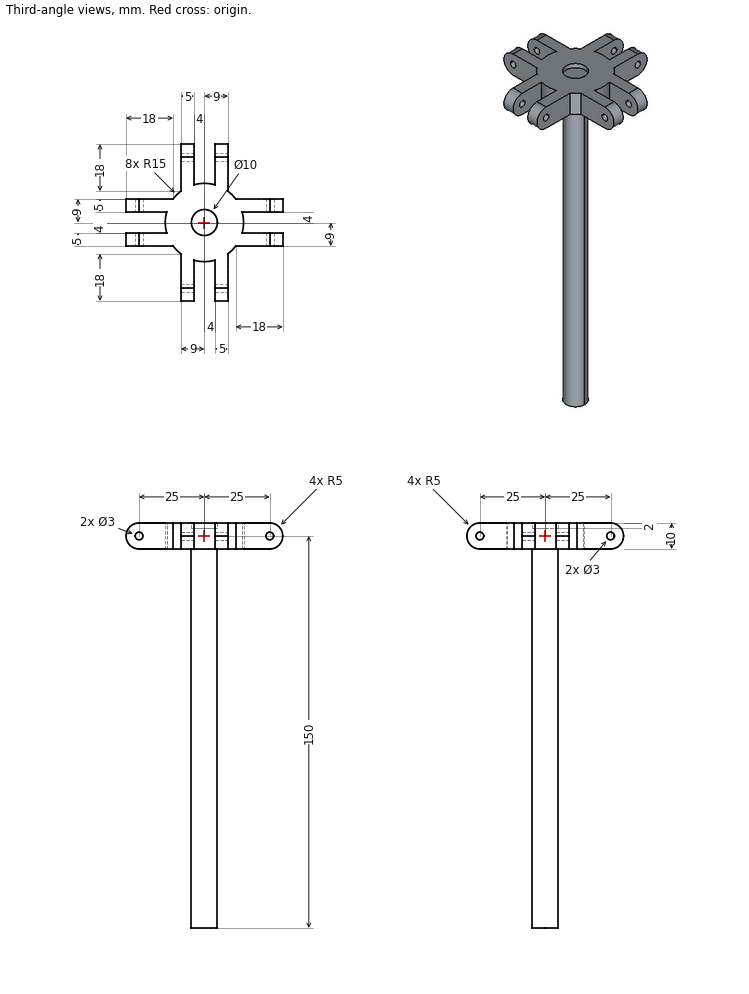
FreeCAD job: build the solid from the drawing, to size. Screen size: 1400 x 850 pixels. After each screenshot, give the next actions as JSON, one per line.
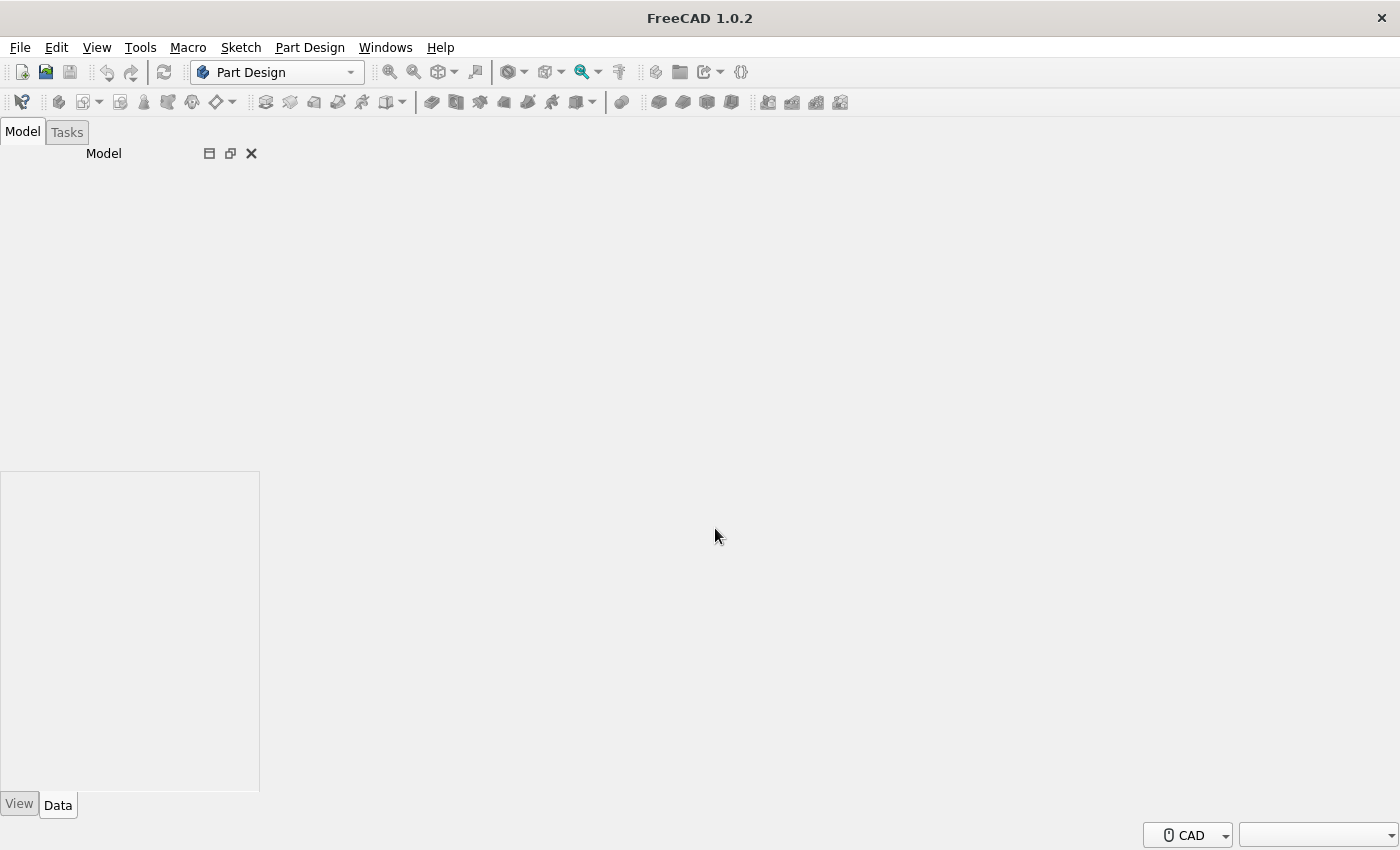
{"action": "left_click", "coordinate": [22, 72]}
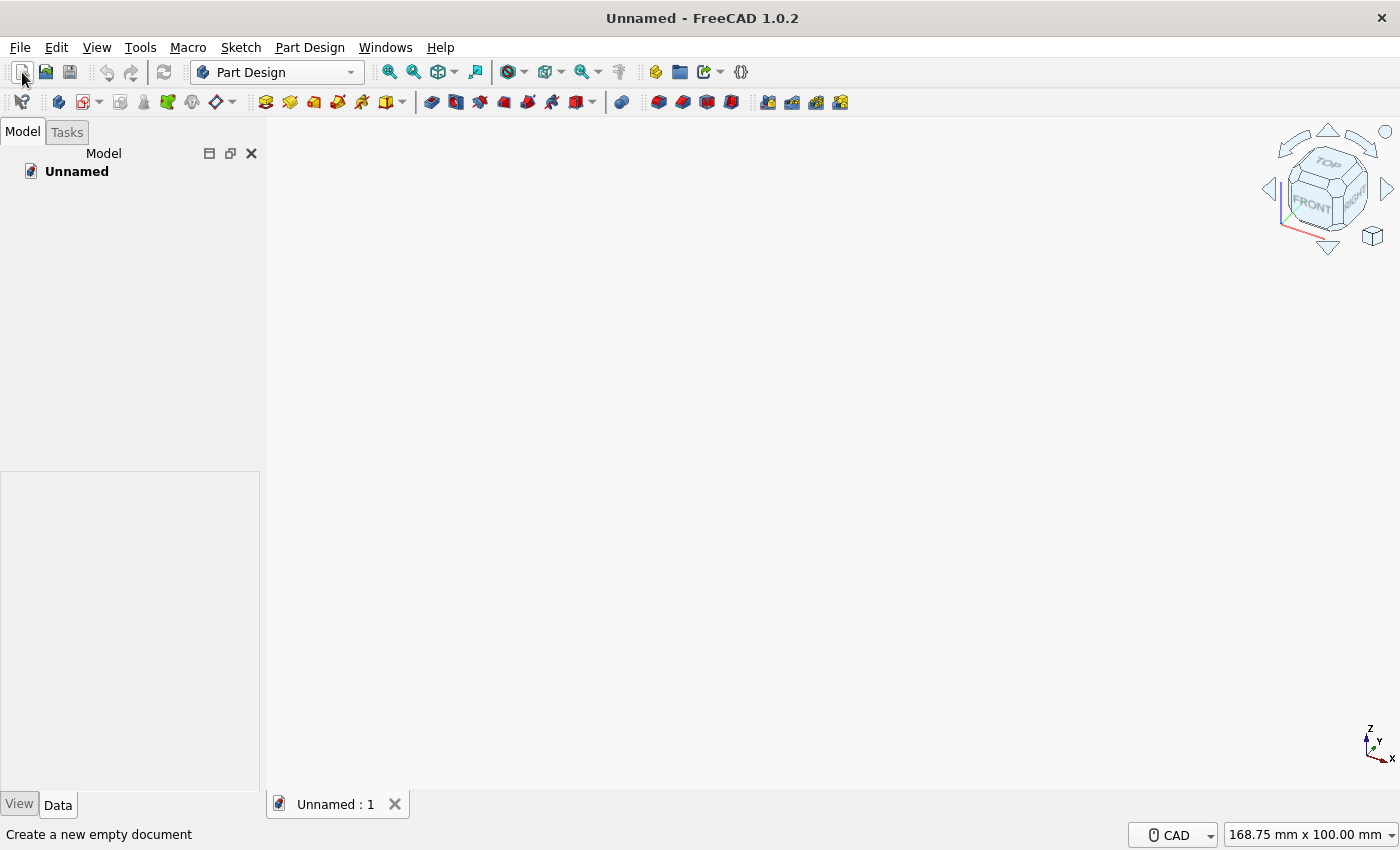
{"action": "left_click", "coordinate": [84, 102]}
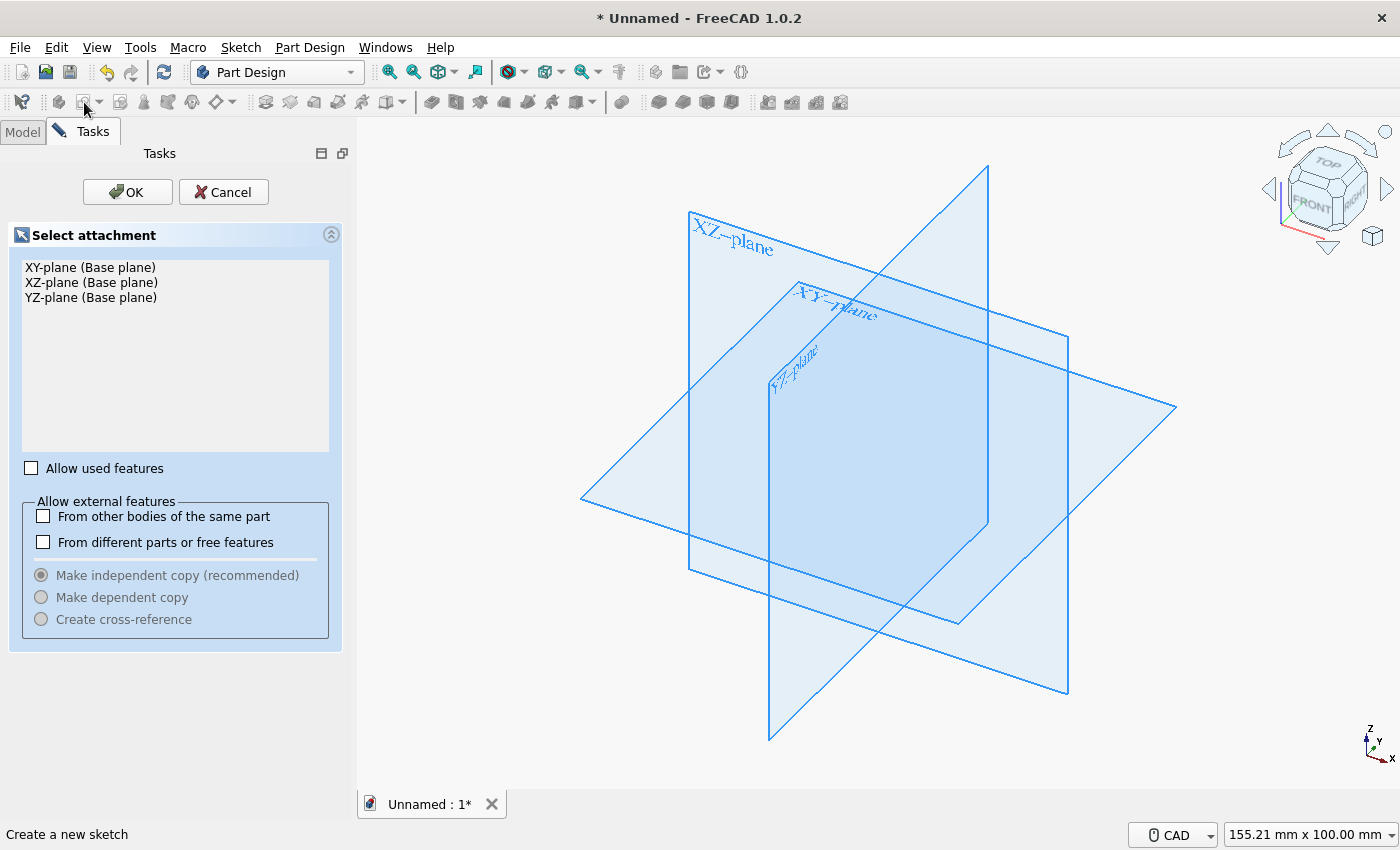
{"action": "left_click", "coordinate": [82, 268]}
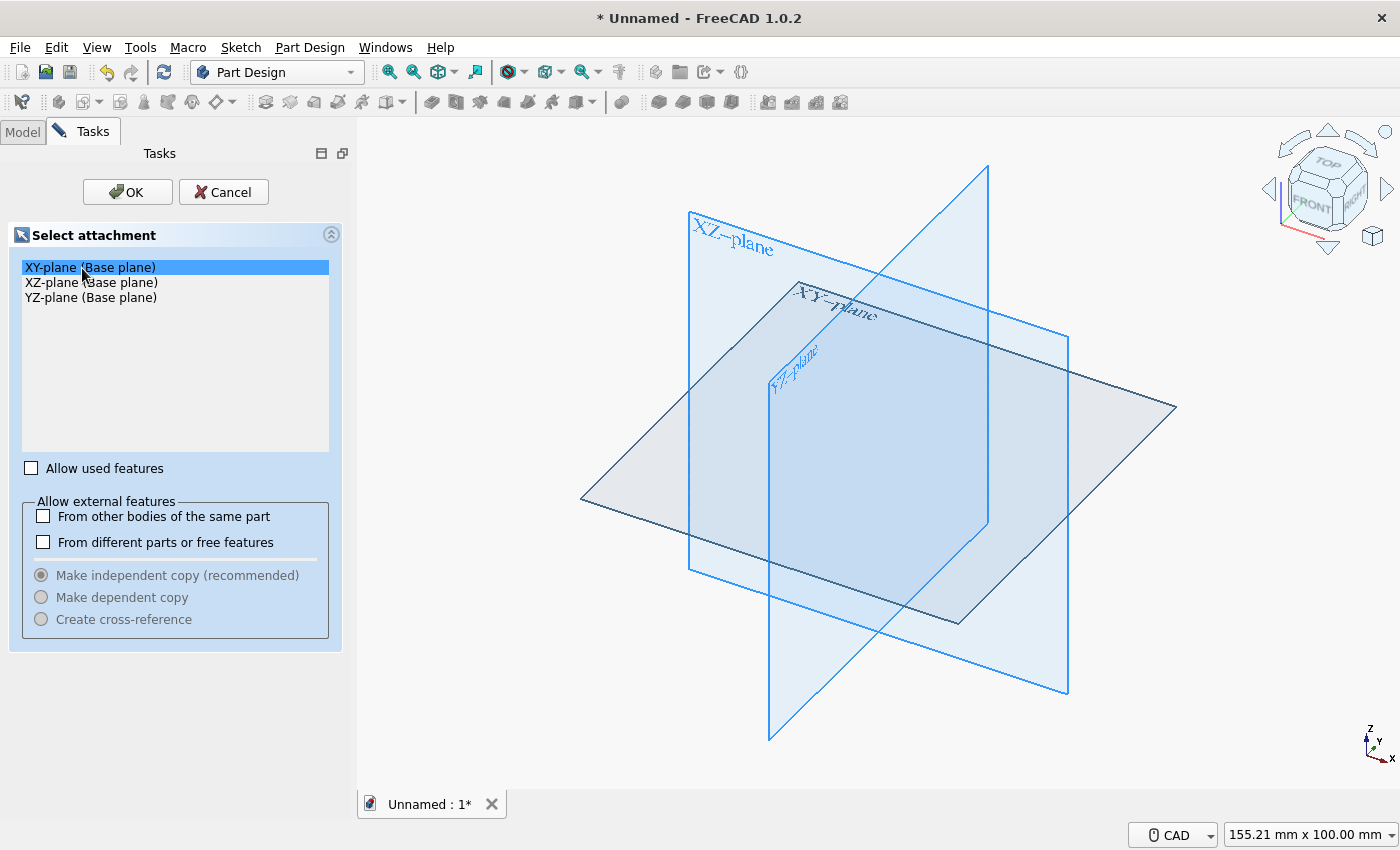
{"action": "left_click", "coordinate": [128, 192]}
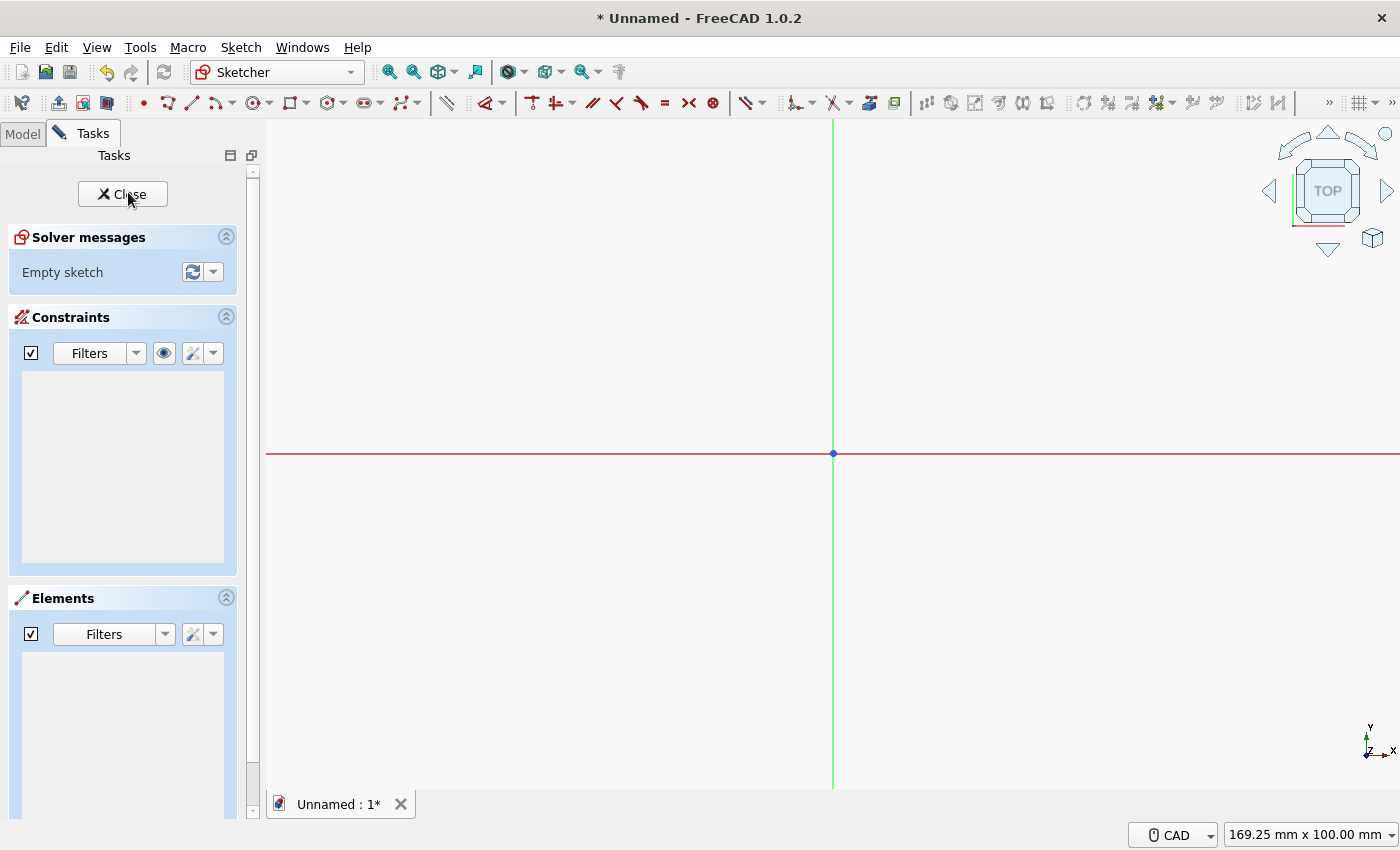
{"action": "key", "text": "g m"}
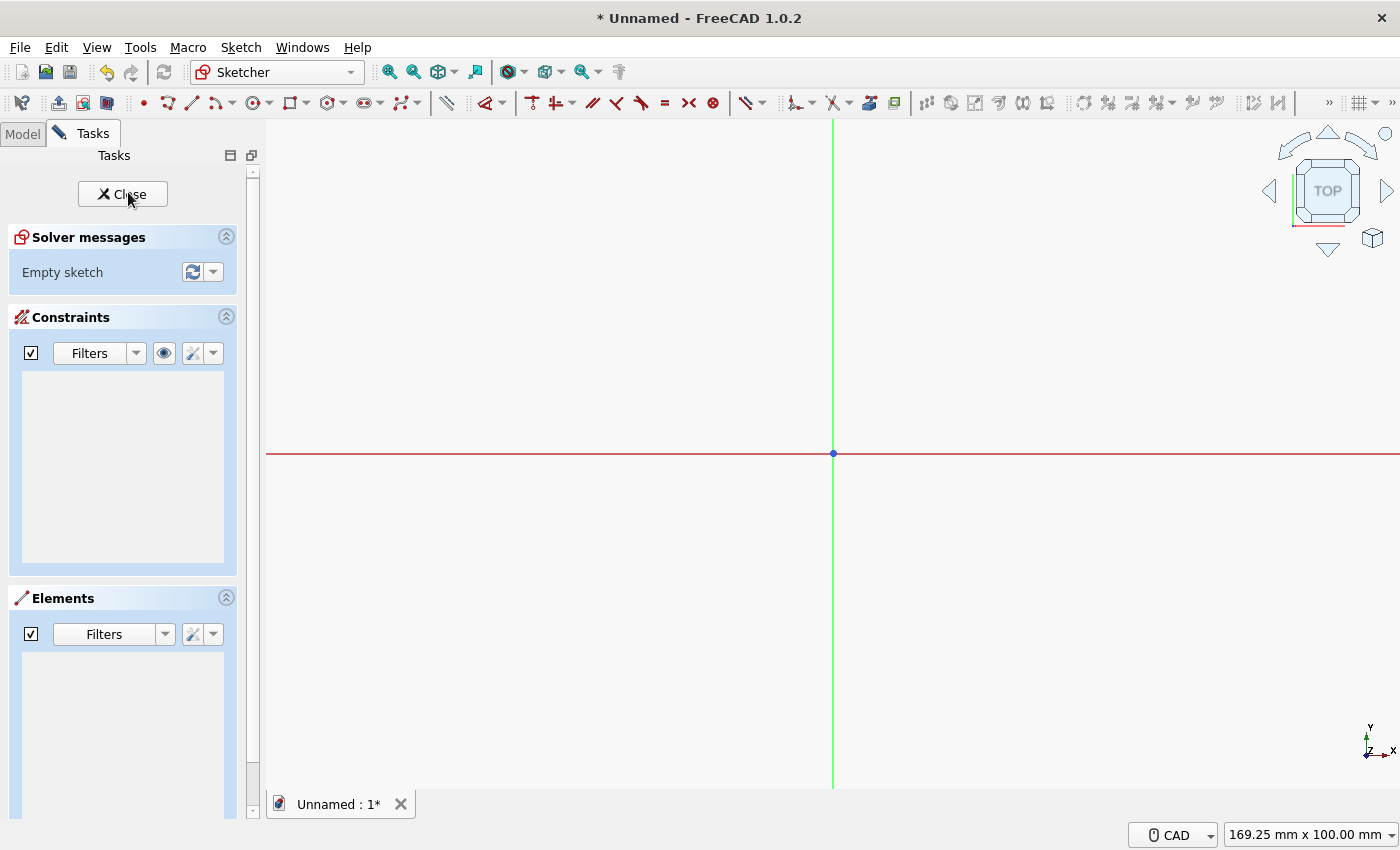
{"action": "left_click", "coordinate": [806, 357]}
{"action": "left_click", "coordinate": [806, 253]}
{"action": "left_click", "coordinate": [773, 253]}
{"action": "left_click", "coordinate": [773, 374]}
{"action": "right_click", "coordinate": [773, 374]}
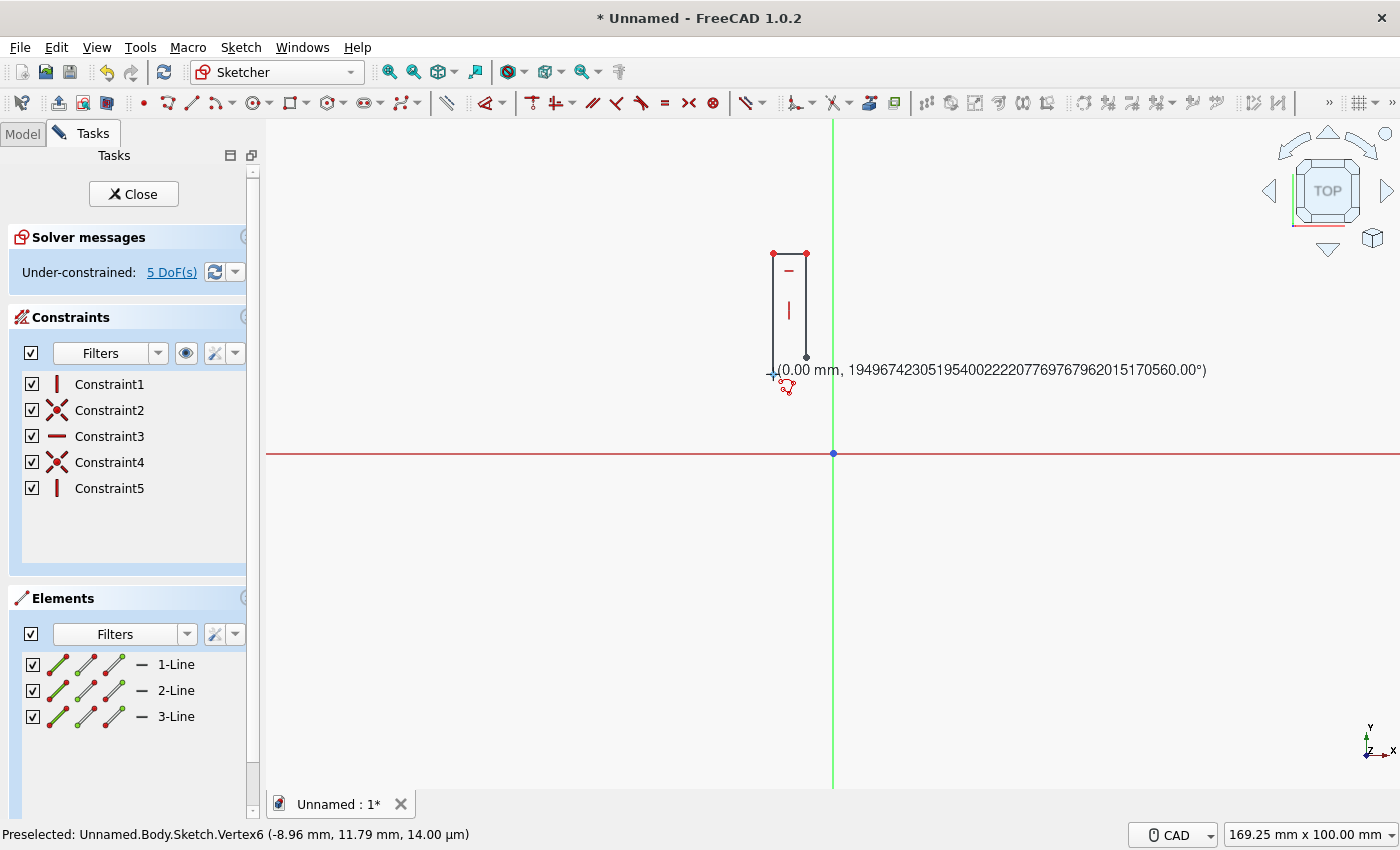
{"action": "left_click", "coordinate": [753, 394]}
{"action": "left_click", "coordinate": [632, 394]}
{"action": "left_click", "coordinate": [632, 427]}
{"action": "left_click", "coordinate": [736, 427]}
{"action": "right_click", "coordinate": [736, 427]}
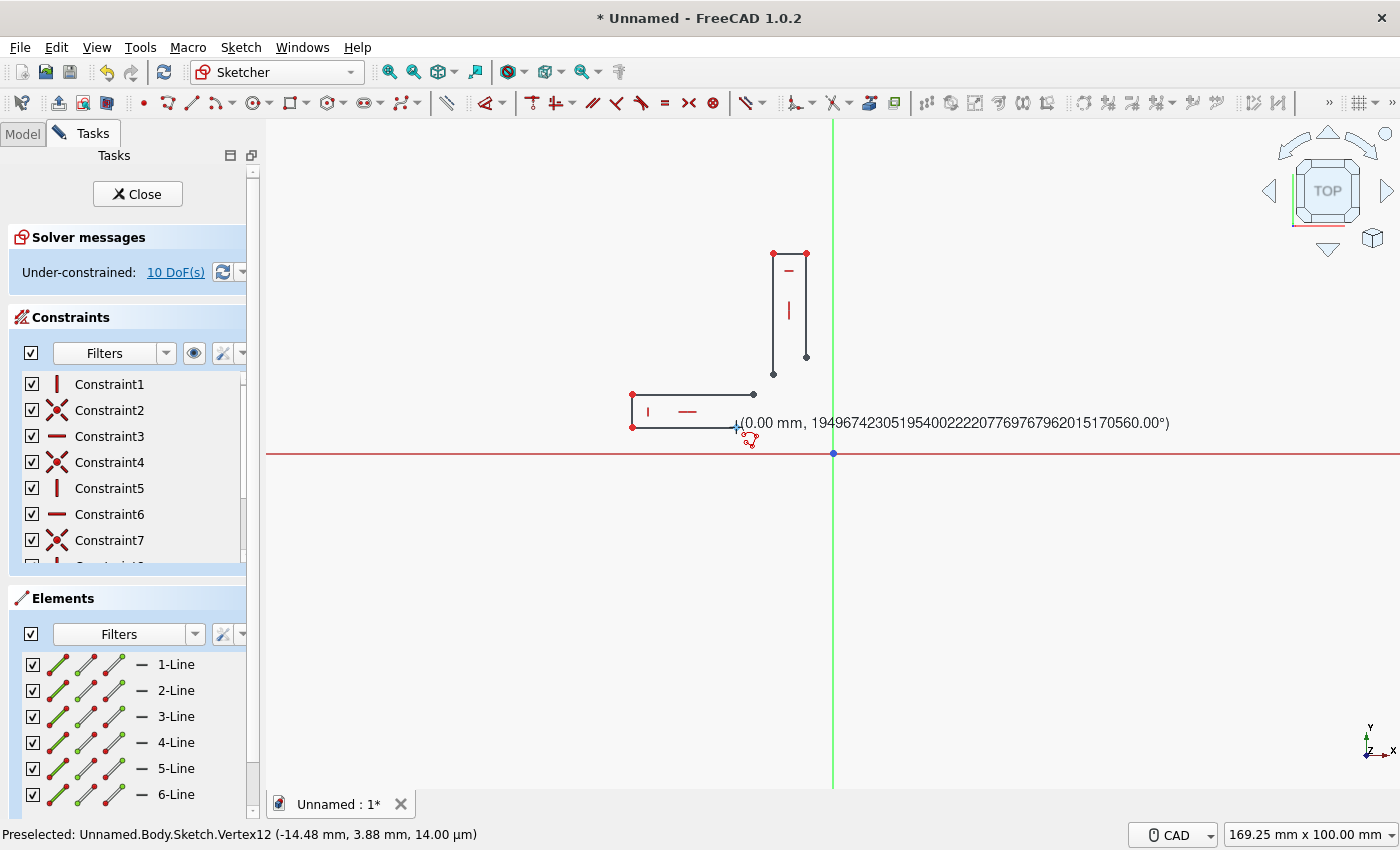
{"action": "left_click", "coordinate": [736, 481]}
{"action": "left_click", "coordinate": [632, 481]}
{"action": "left_click", "coordinate": [632, 514]}
{"action": "left_click", "coordinate": [753, 514]}
{"action": "right_click", "coordinate": [753, 514]}